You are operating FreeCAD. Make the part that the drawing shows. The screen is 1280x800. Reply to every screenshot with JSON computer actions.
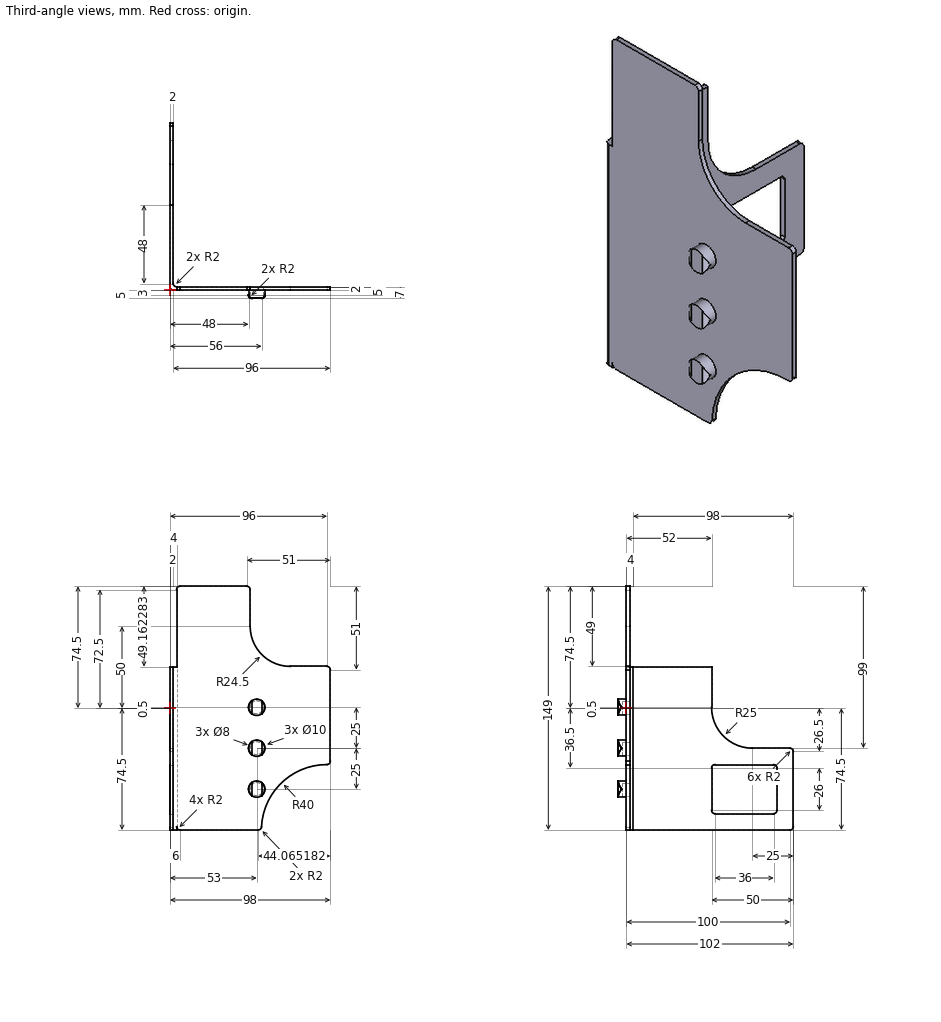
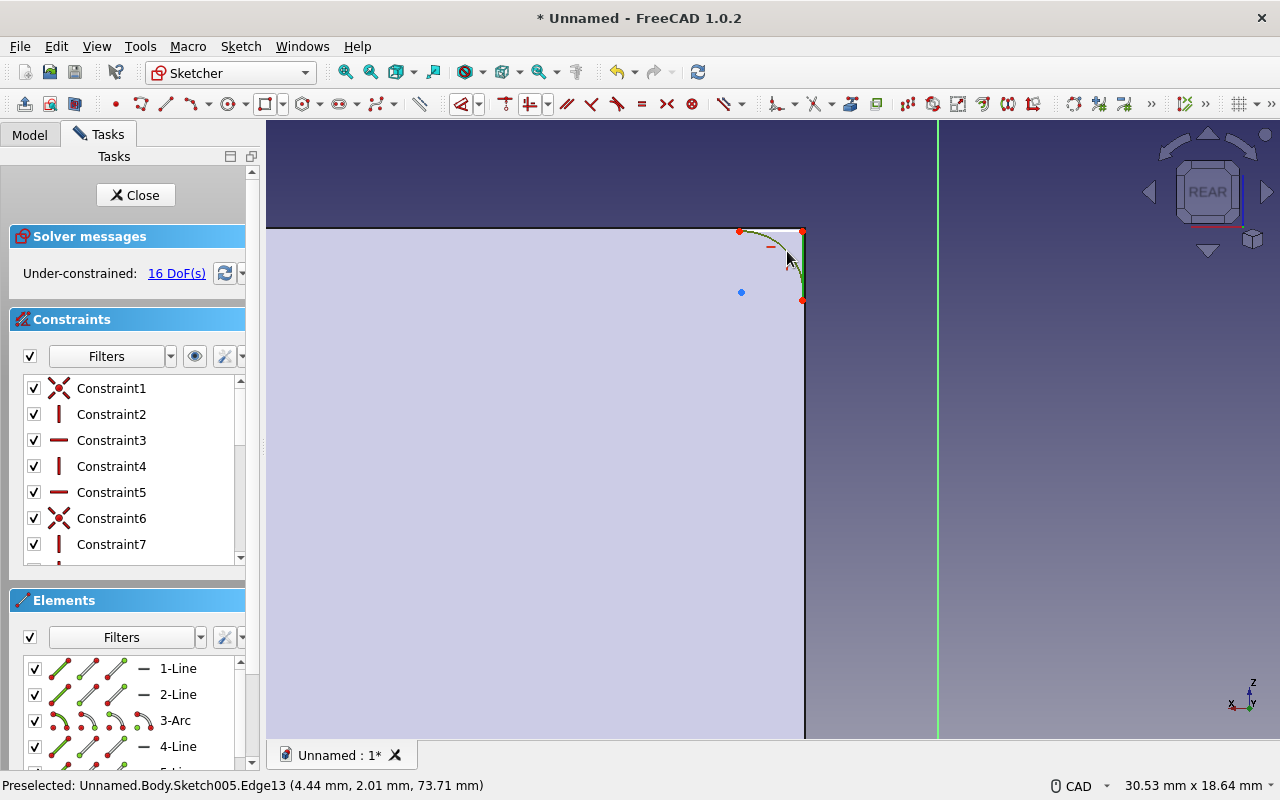
{"action": "key", "text": "t"}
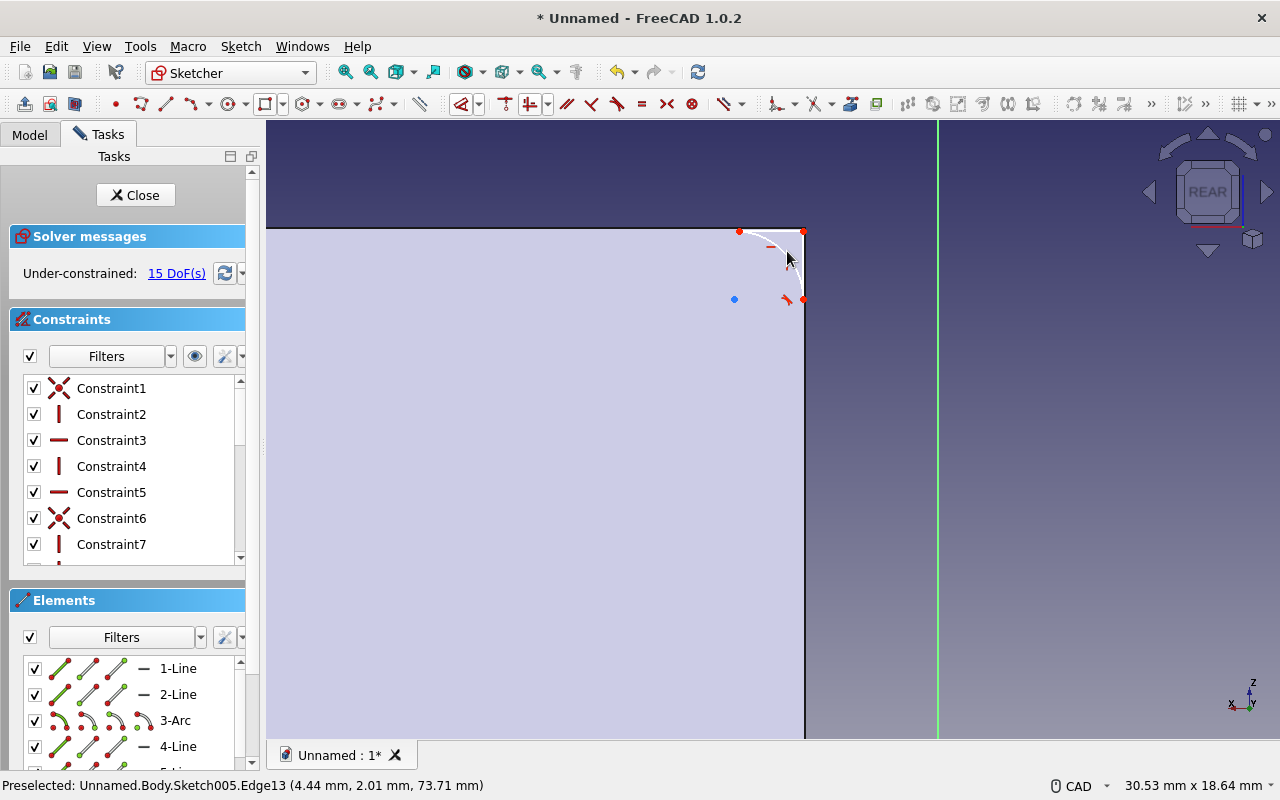
{"action": "left_click", "coordinate": [784, 231]}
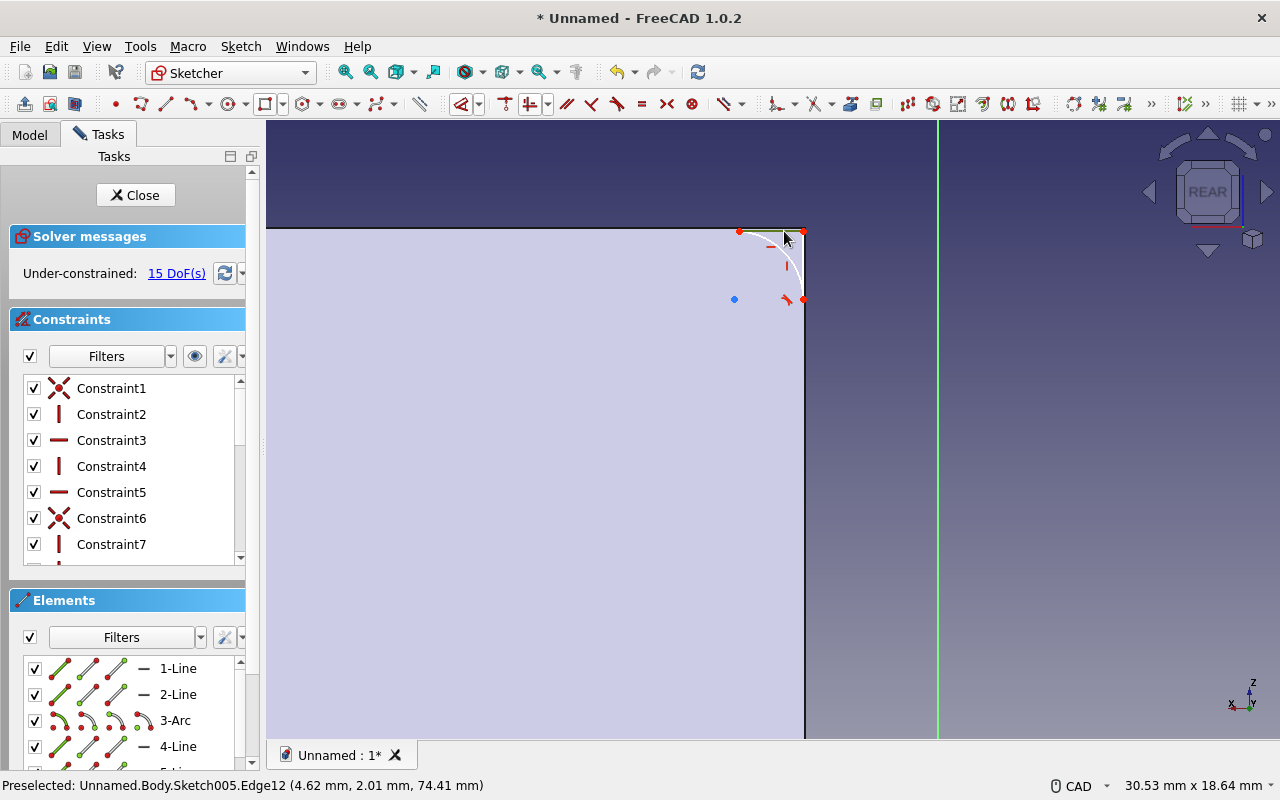
{"action": "scroll", "coordinate": [769, 240], "scroll_direction": "up", "scroll_amount": 2}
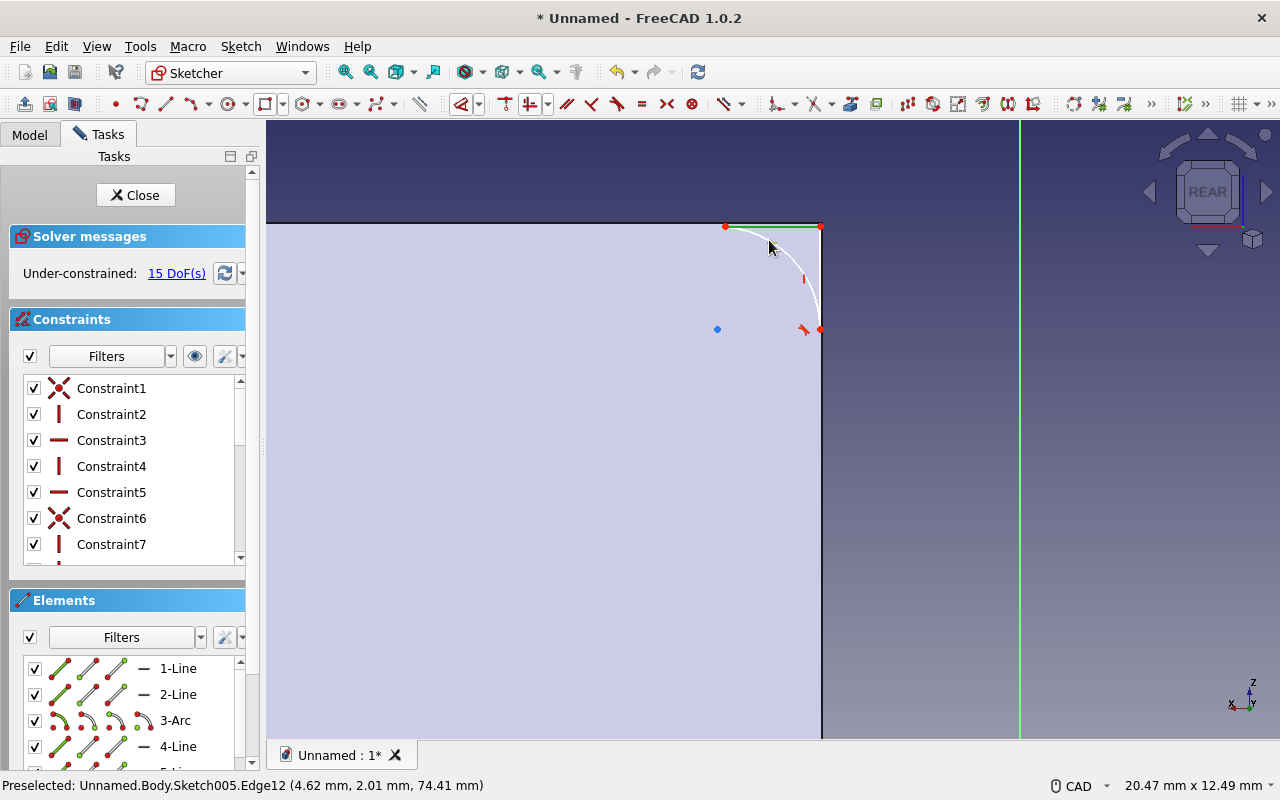
{"action": "left_click", "coordinate": [793, 260]}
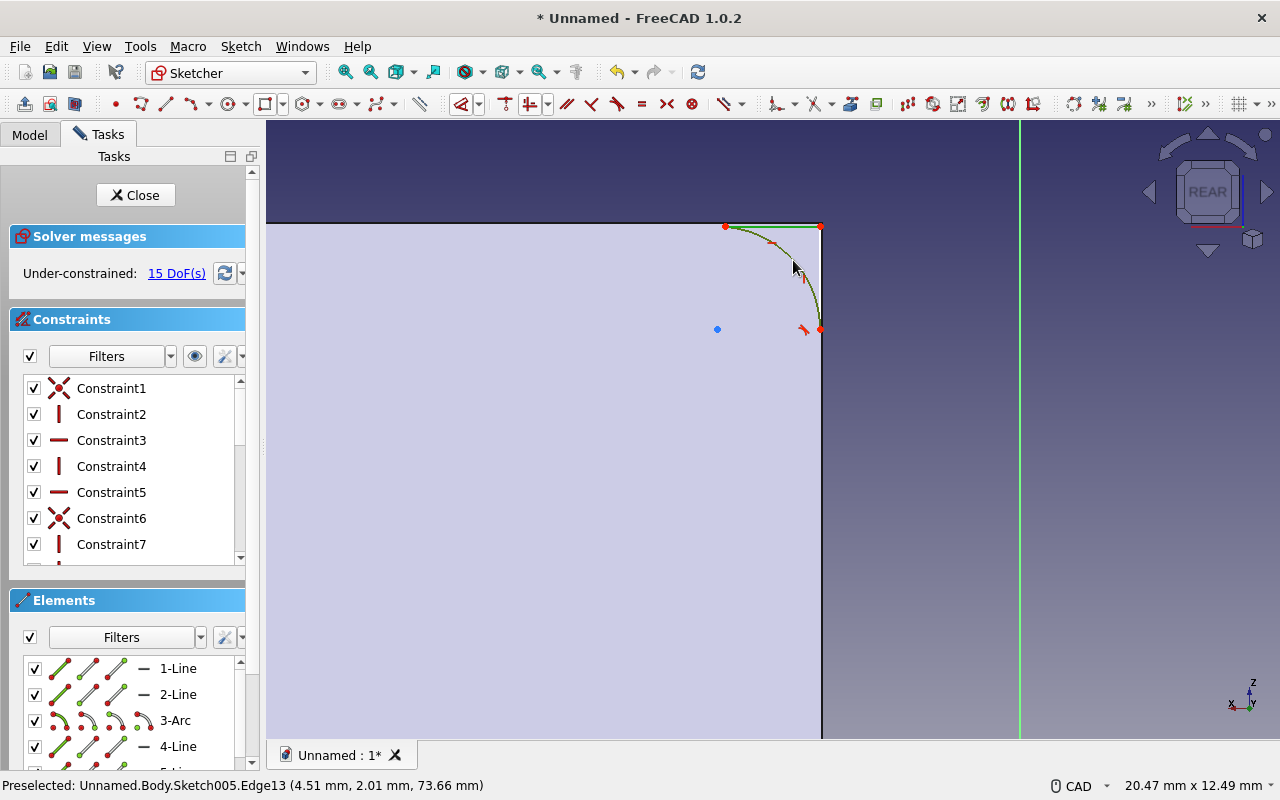
{"action": "left_click", "coordinate": [617, 104]}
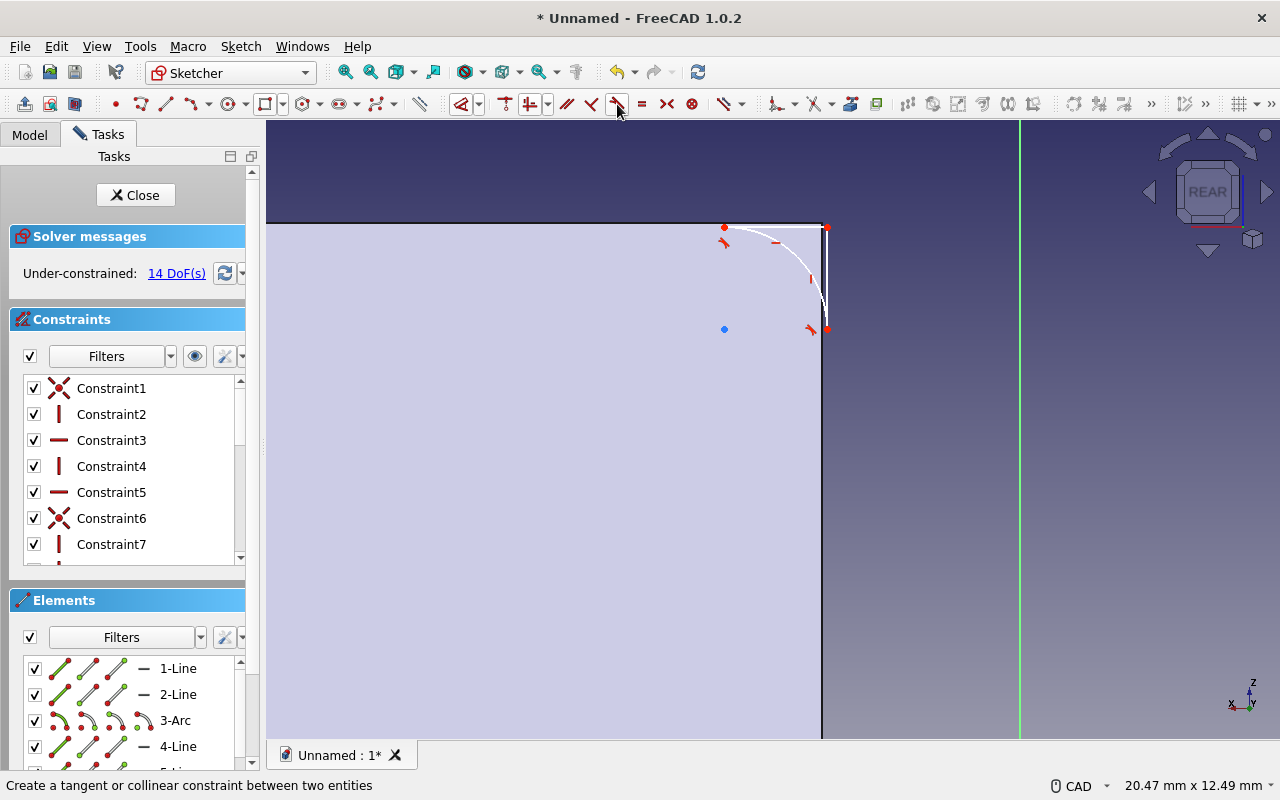
{"action": "scroll", "coordinate": [815, 247], "scroll_direction": "down", "scroll_amount": 15}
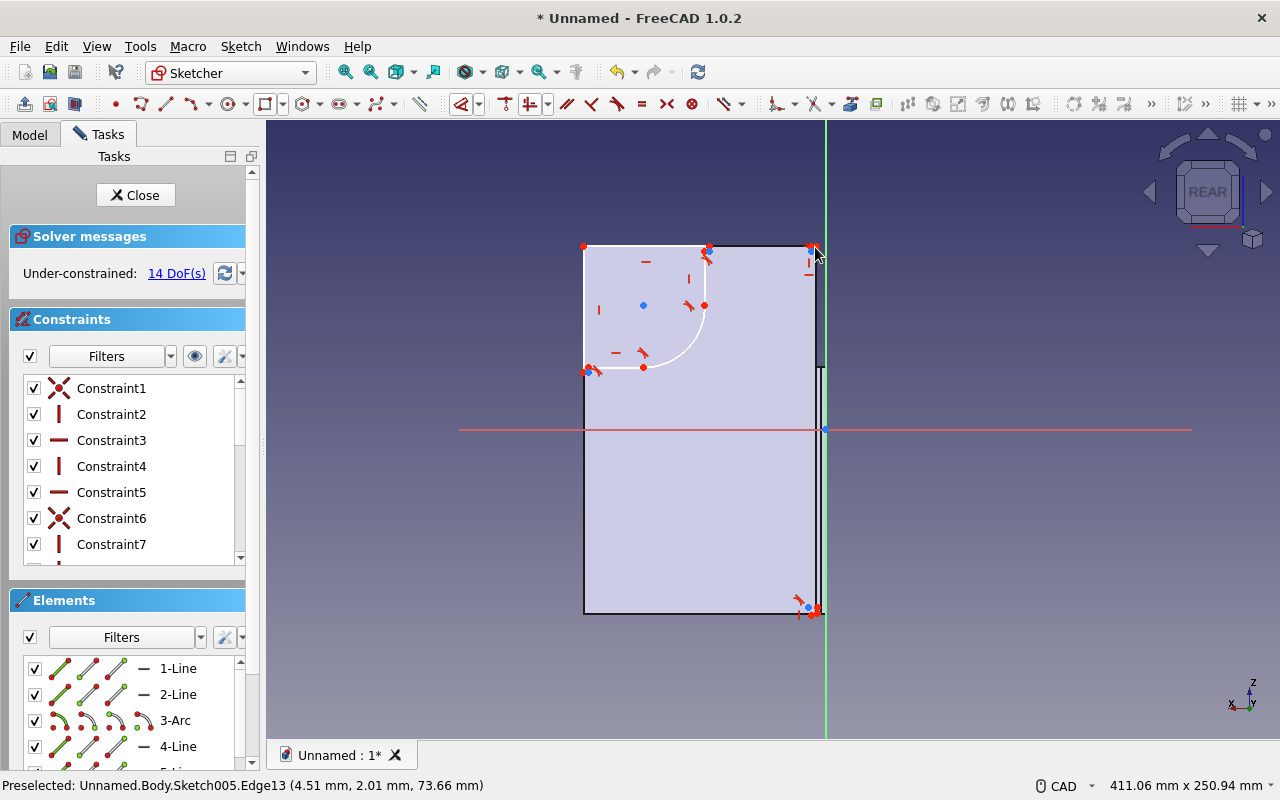
{"action": "scroll", "coordinate": [815, 614], "scroll_direction": "up", "scroll_amount": 13}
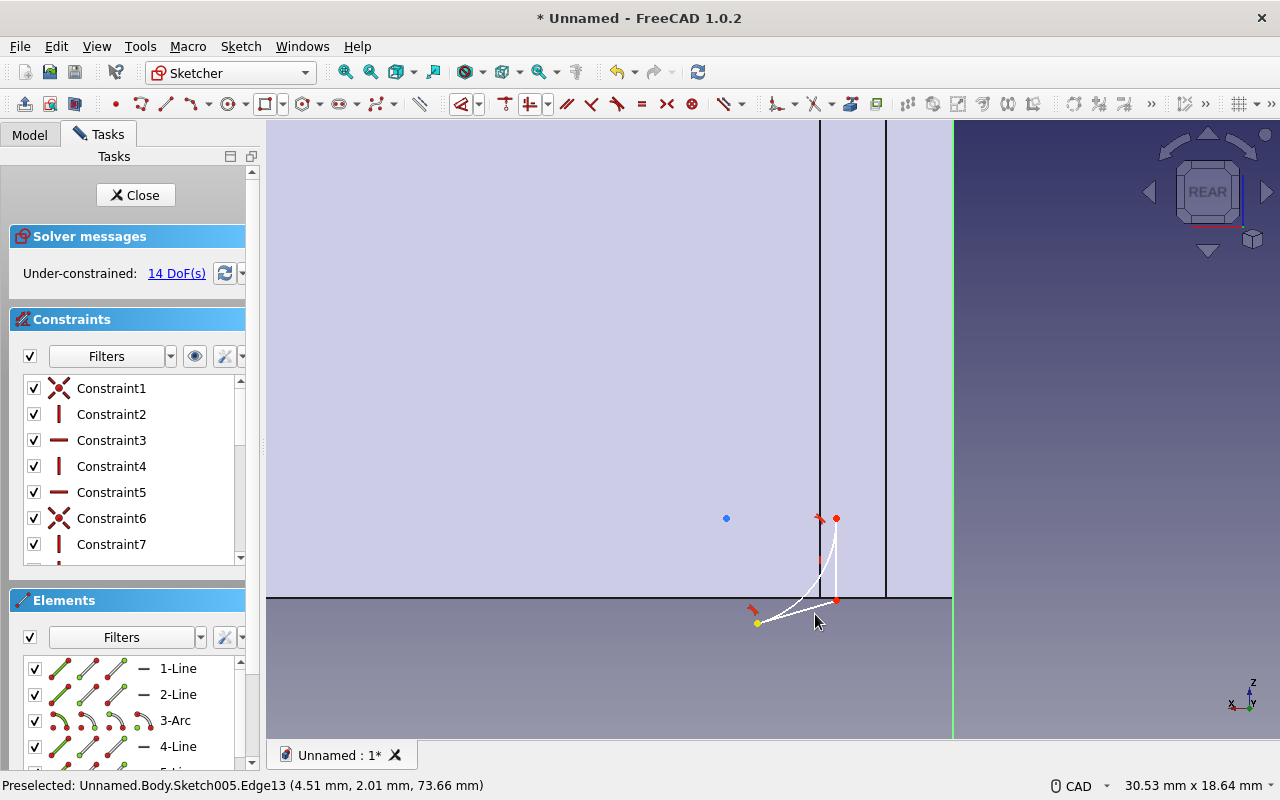
{"action": "left_click", "coordinate": [813, 608]}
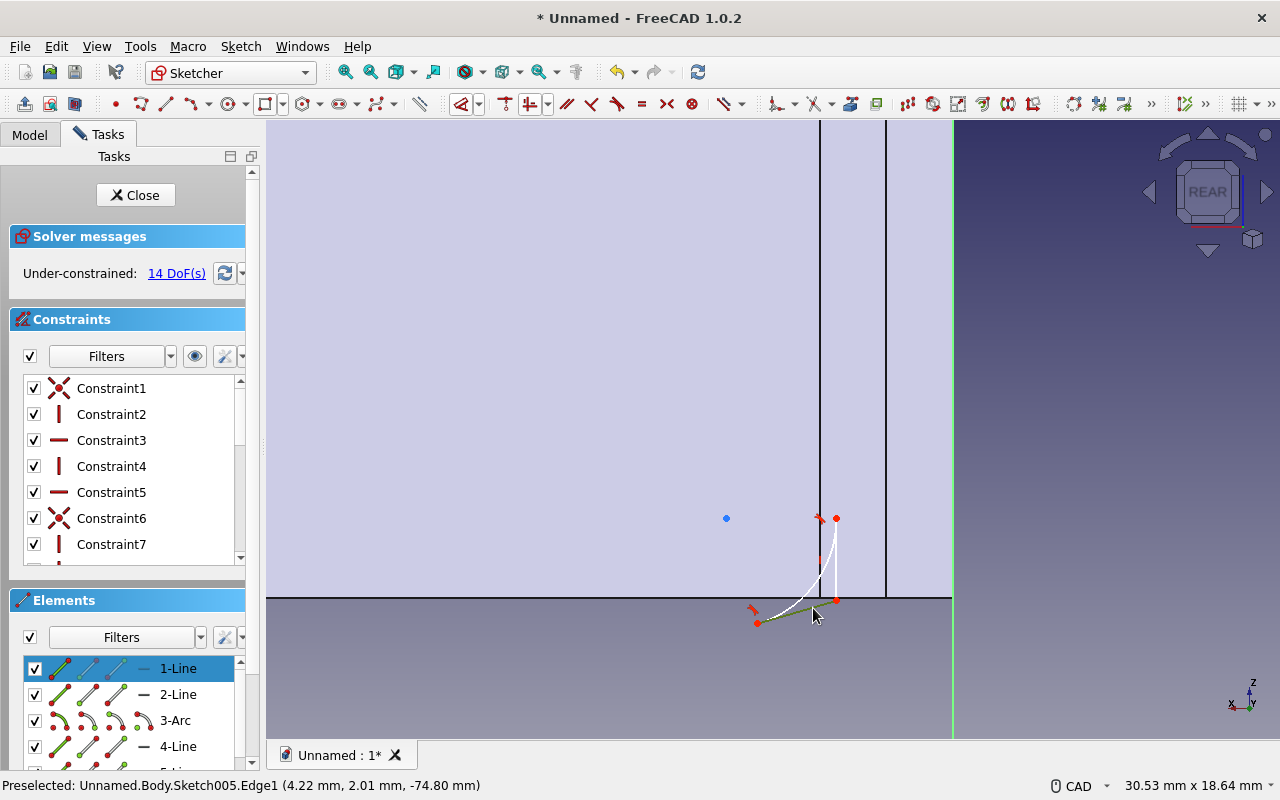
{"action": "key", "text": "h"}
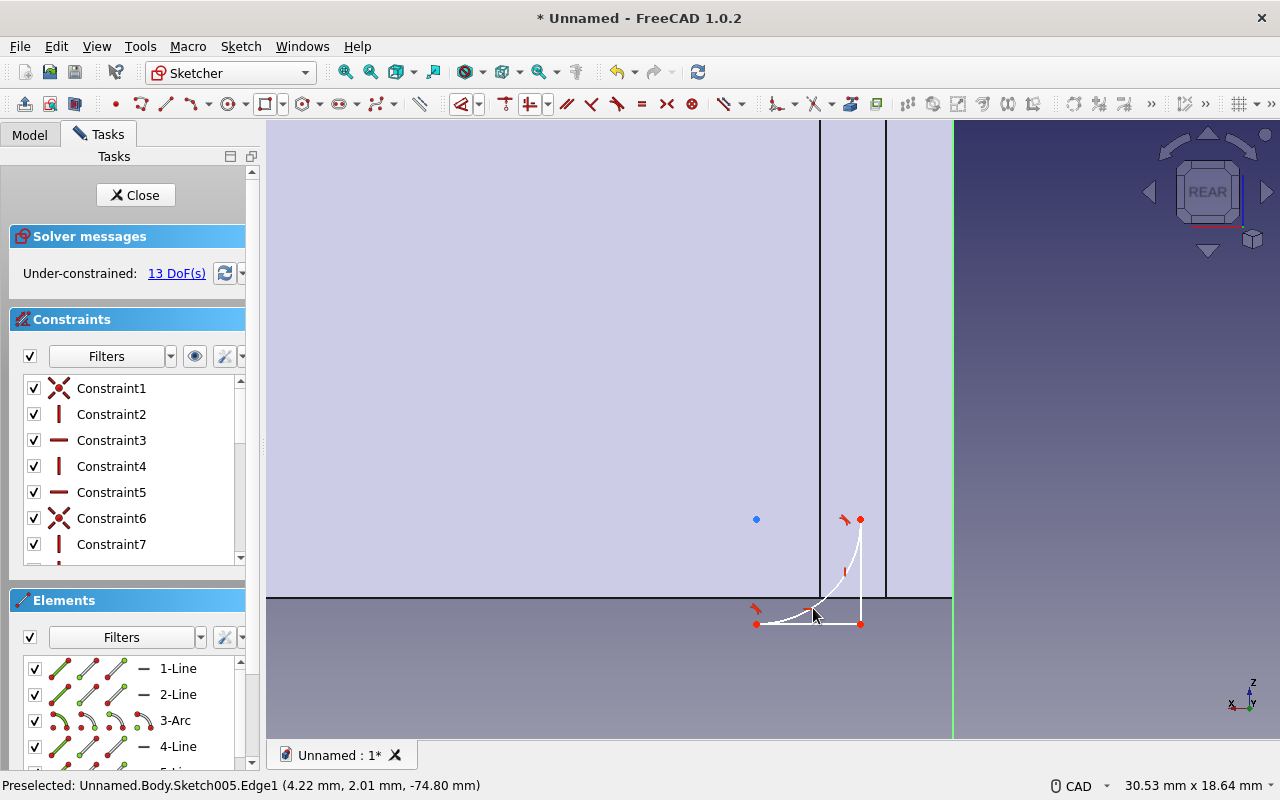
{"action": "left_click", "coordinate": [830, 594]}